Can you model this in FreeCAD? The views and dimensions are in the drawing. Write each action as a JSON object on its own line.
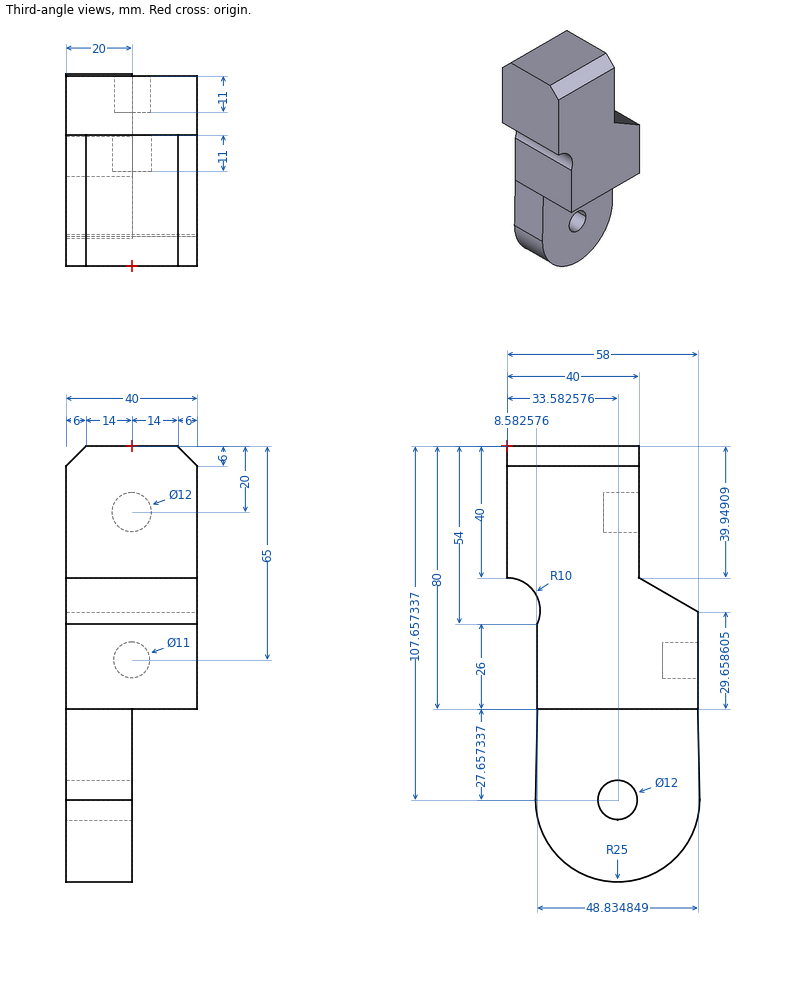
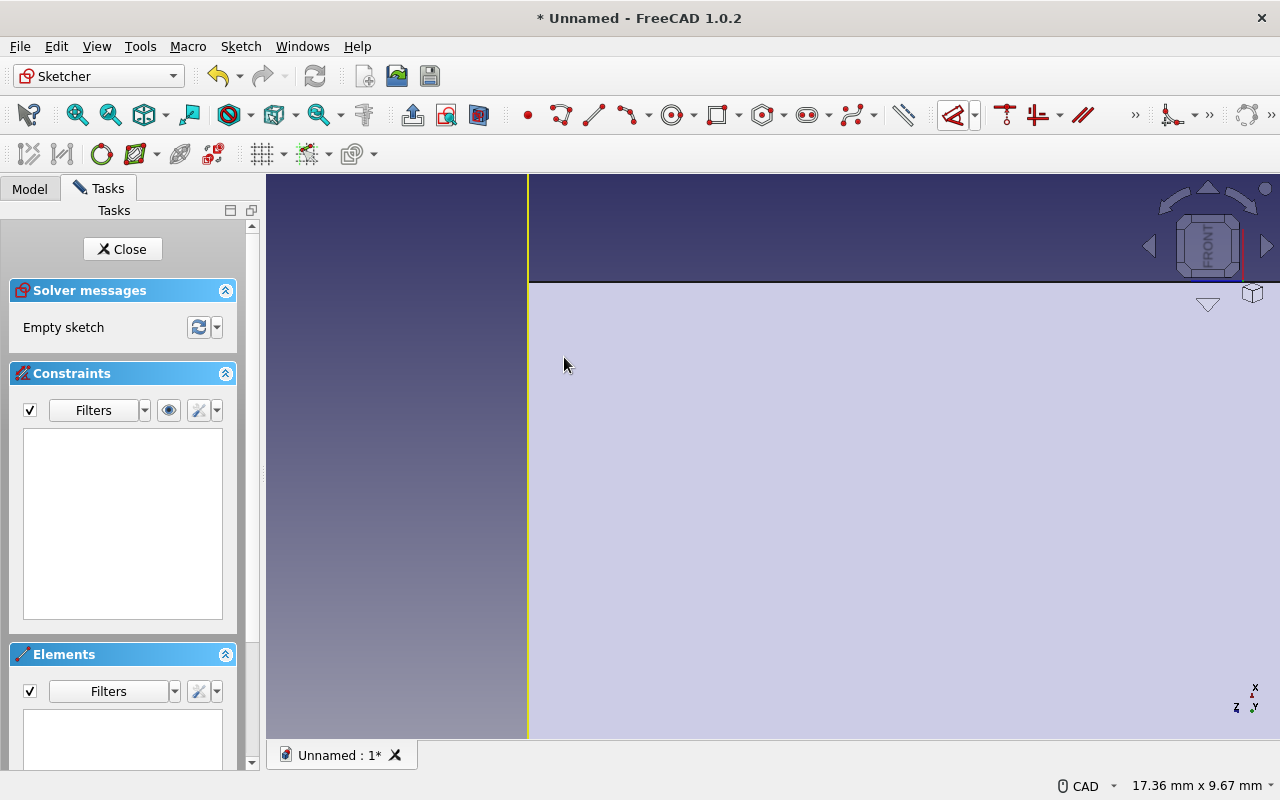
{"action": "left_click", "coordinate": [561, 116]}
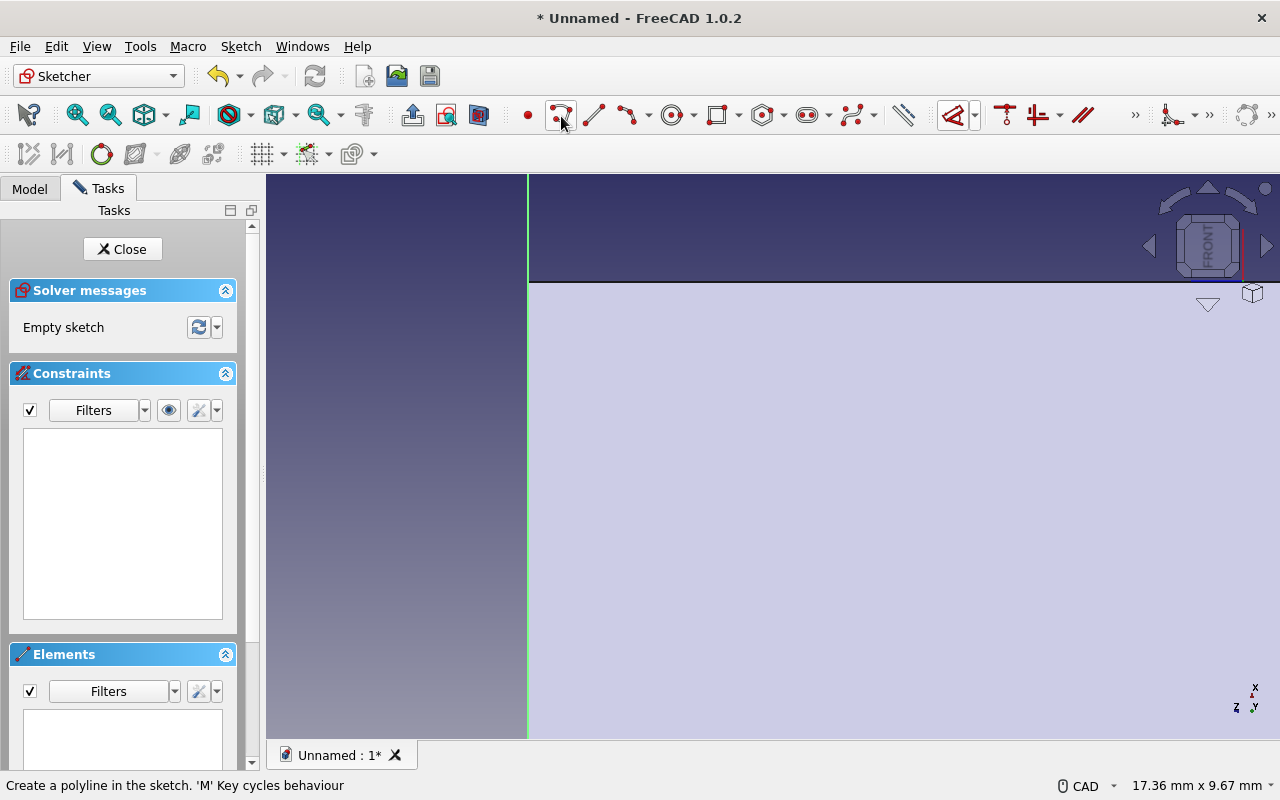
{"action": "left_click", "coordinate": [528, 633]}
{"action": "left_click", "coordinate": [878, 282]}
{"action": "left_click", "coordinate": [537, 282]}
{"action": "left_click", "coordinate": [528, 634]}
{"action": "key", "text": "Escape"}
{"action": "key", "text": "Escape"}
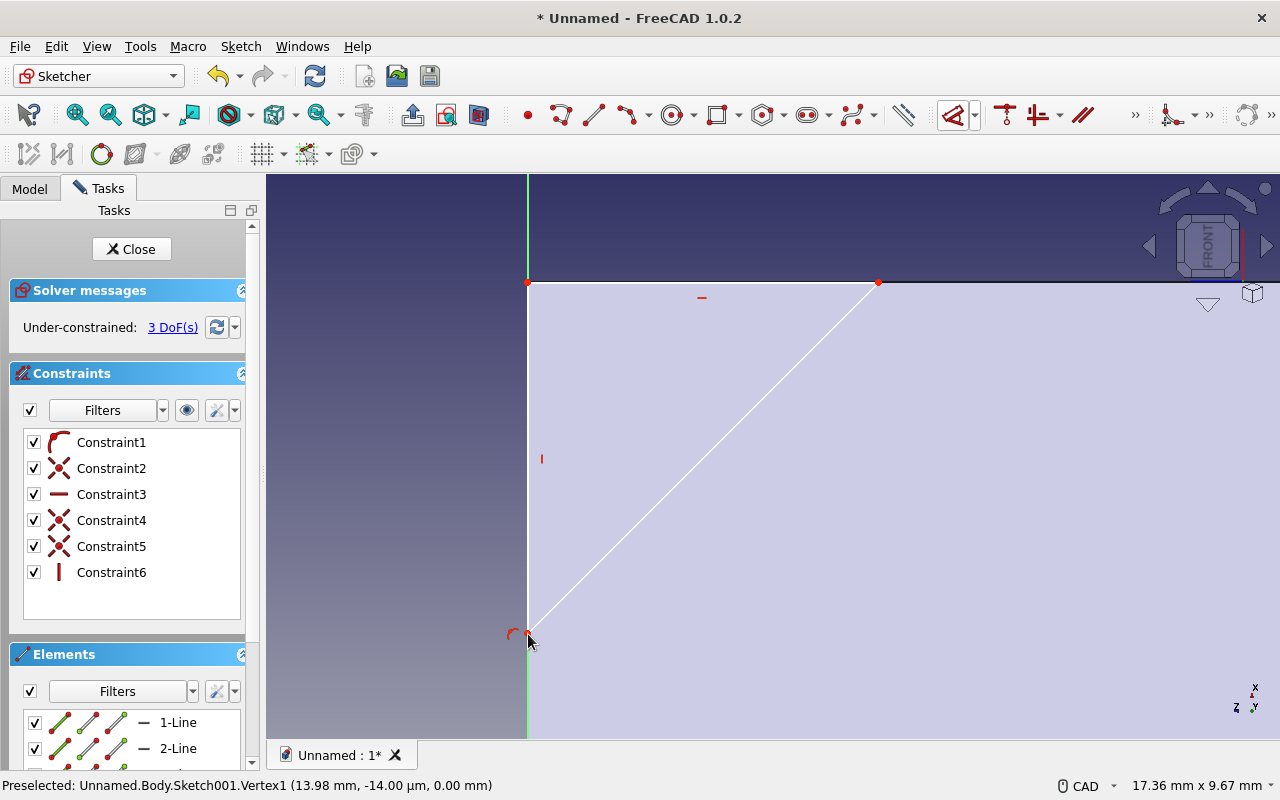
{"action": "left_click", "coordinate": [773, 283]}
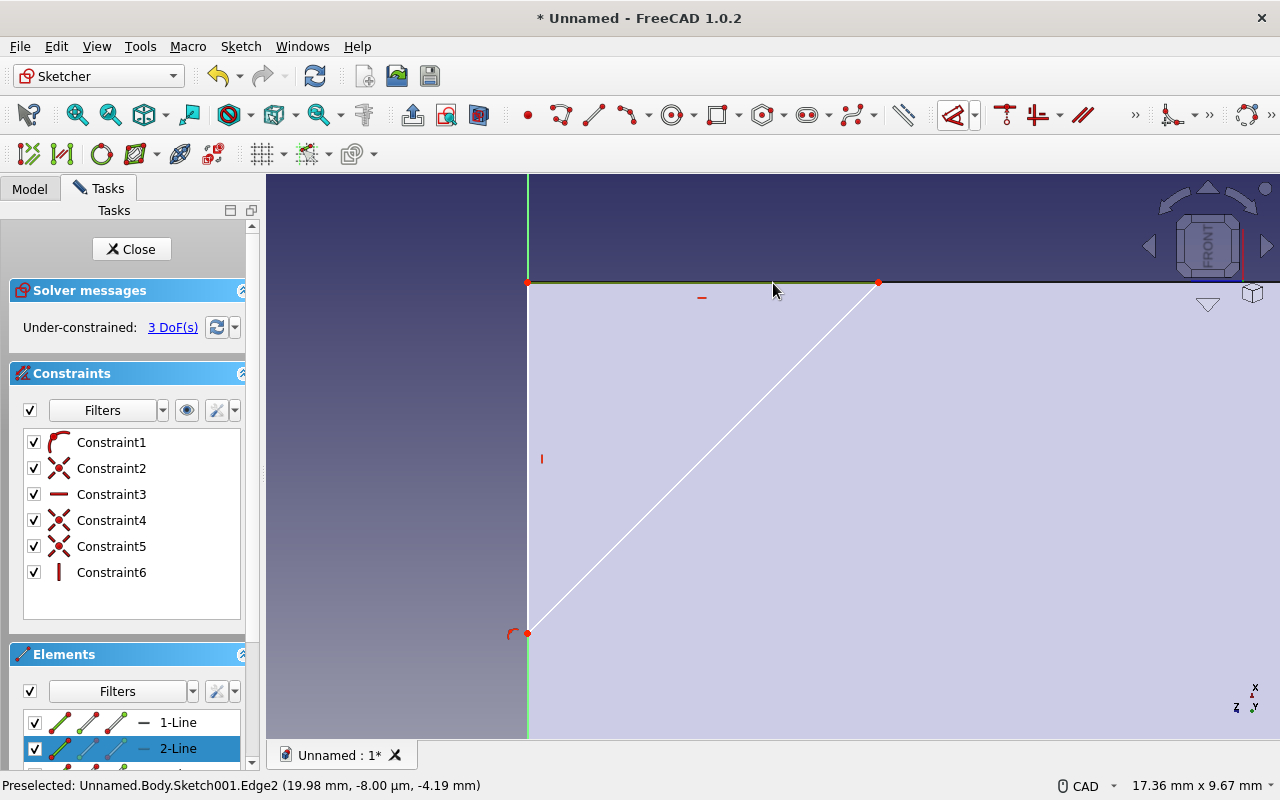
{"action": "key", "text": "l"}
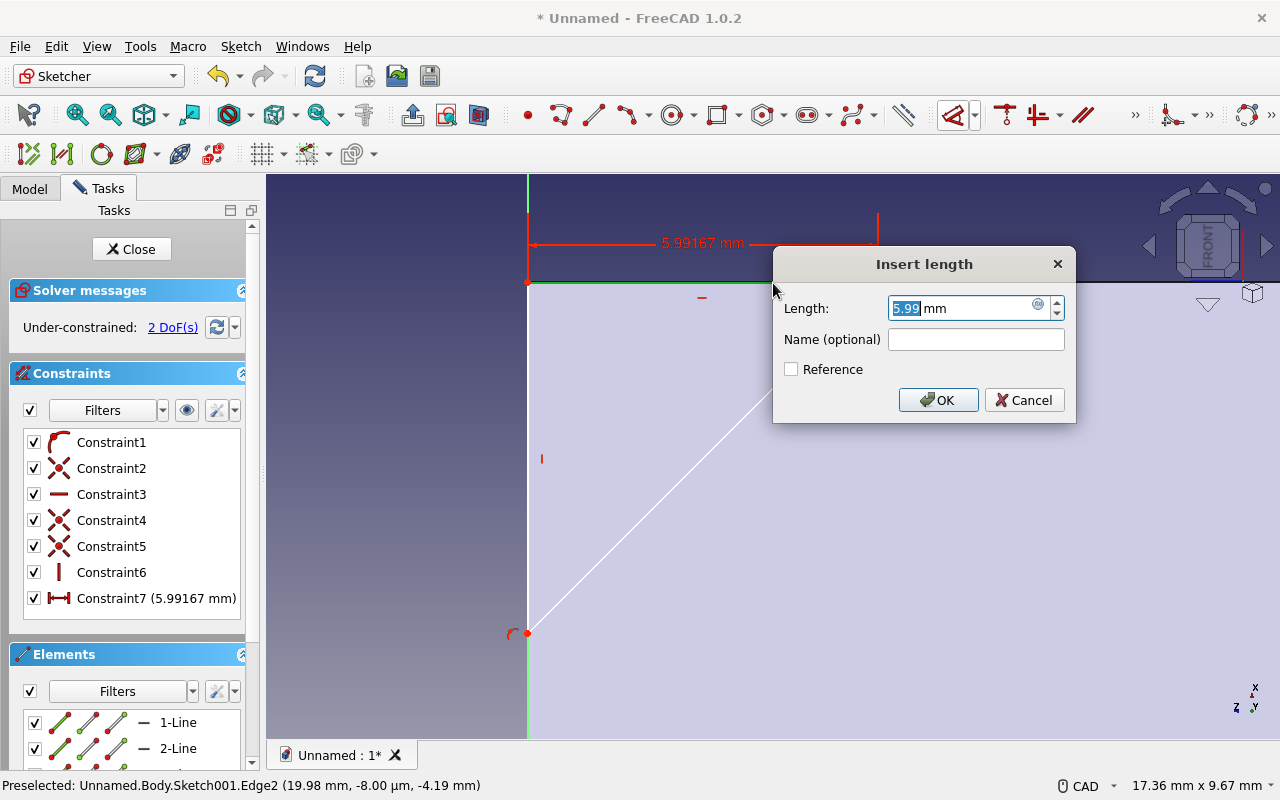
{"action": "type", "text": "6"}
{"action": "key", "text": "Return"}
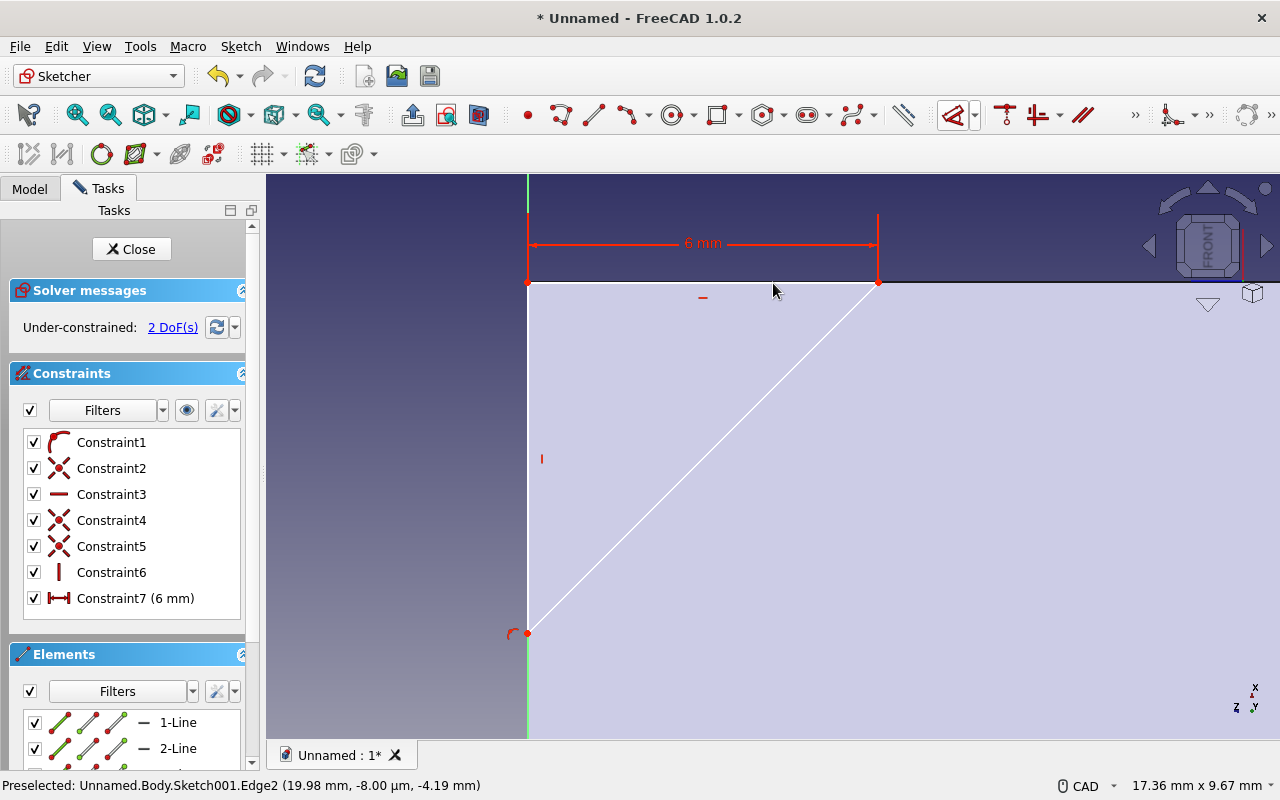
{"action": "left_click", "coordinate": [528, 388]}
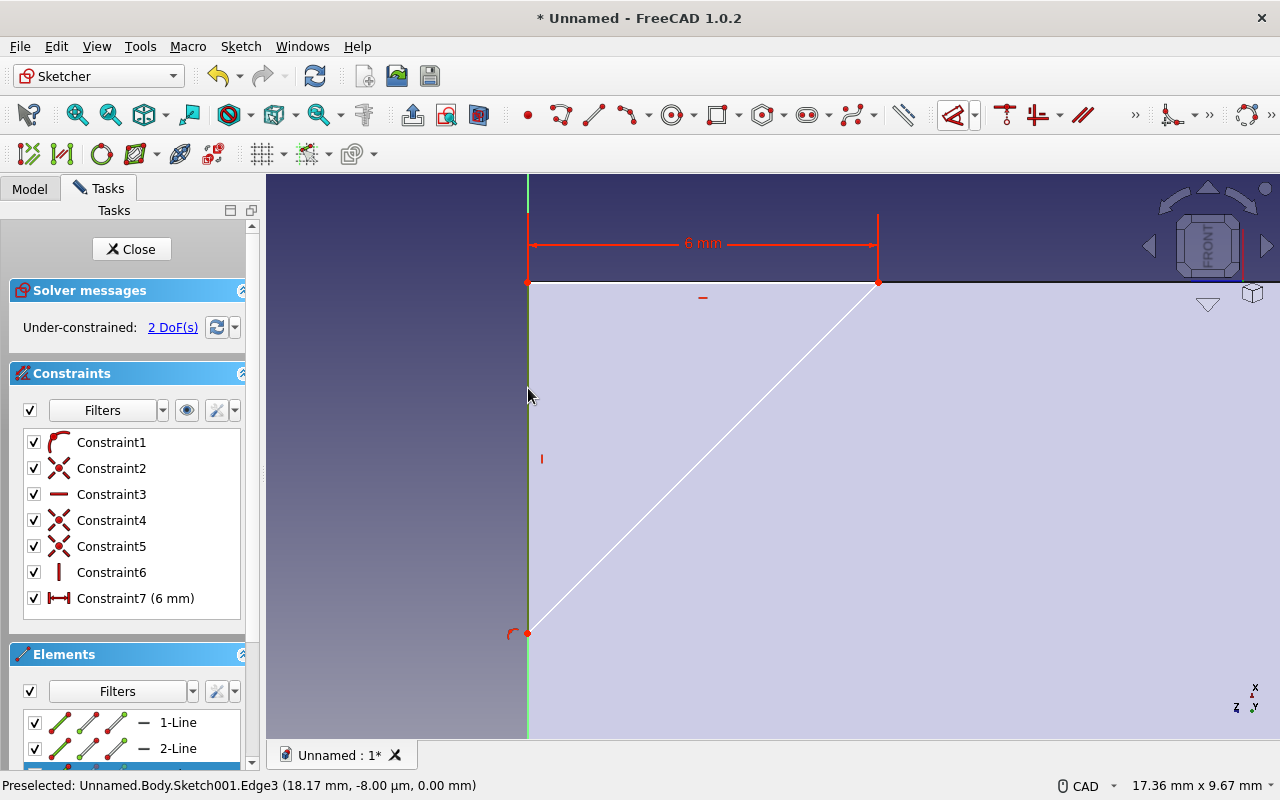
{"action": "key", "text": "i"}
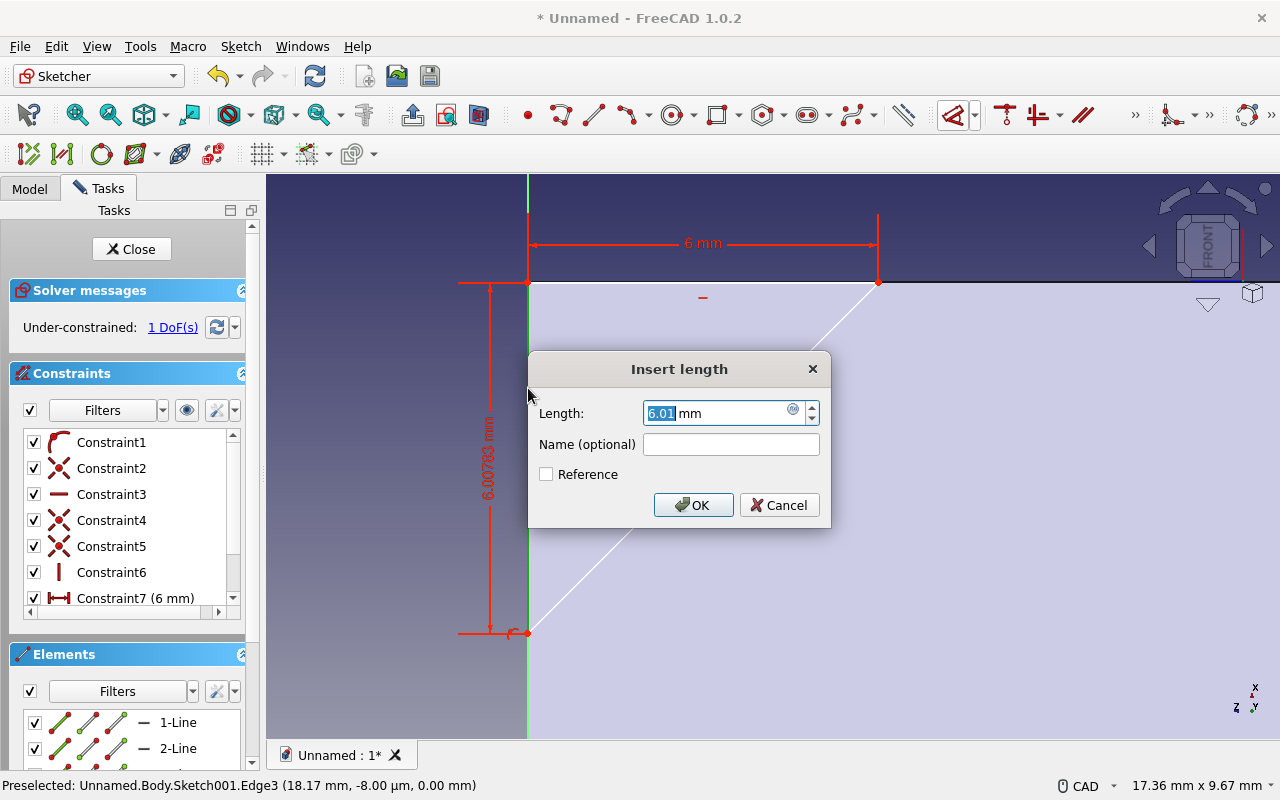
{"action": "type", "text": "6"}
{"action": "key", "text": "Return"}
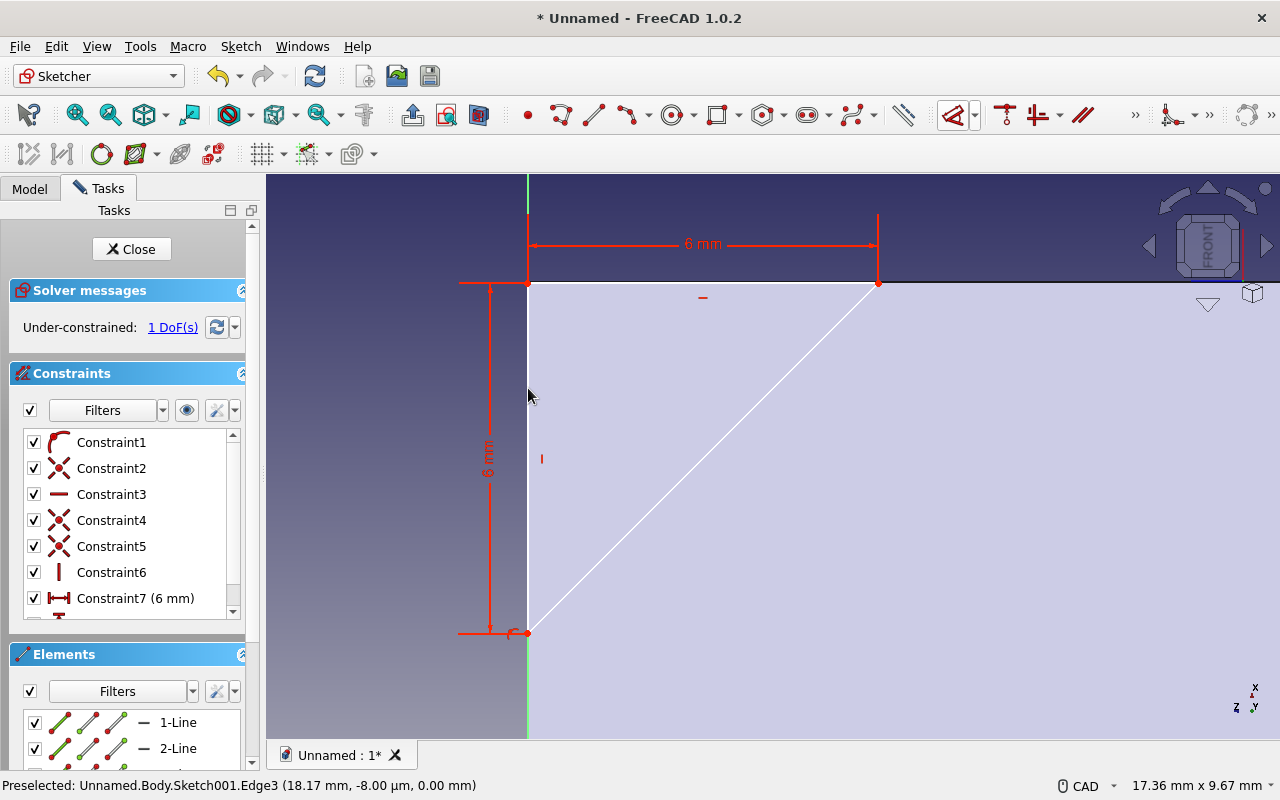
{"action": "left_click", "coordinate": [528, 634]}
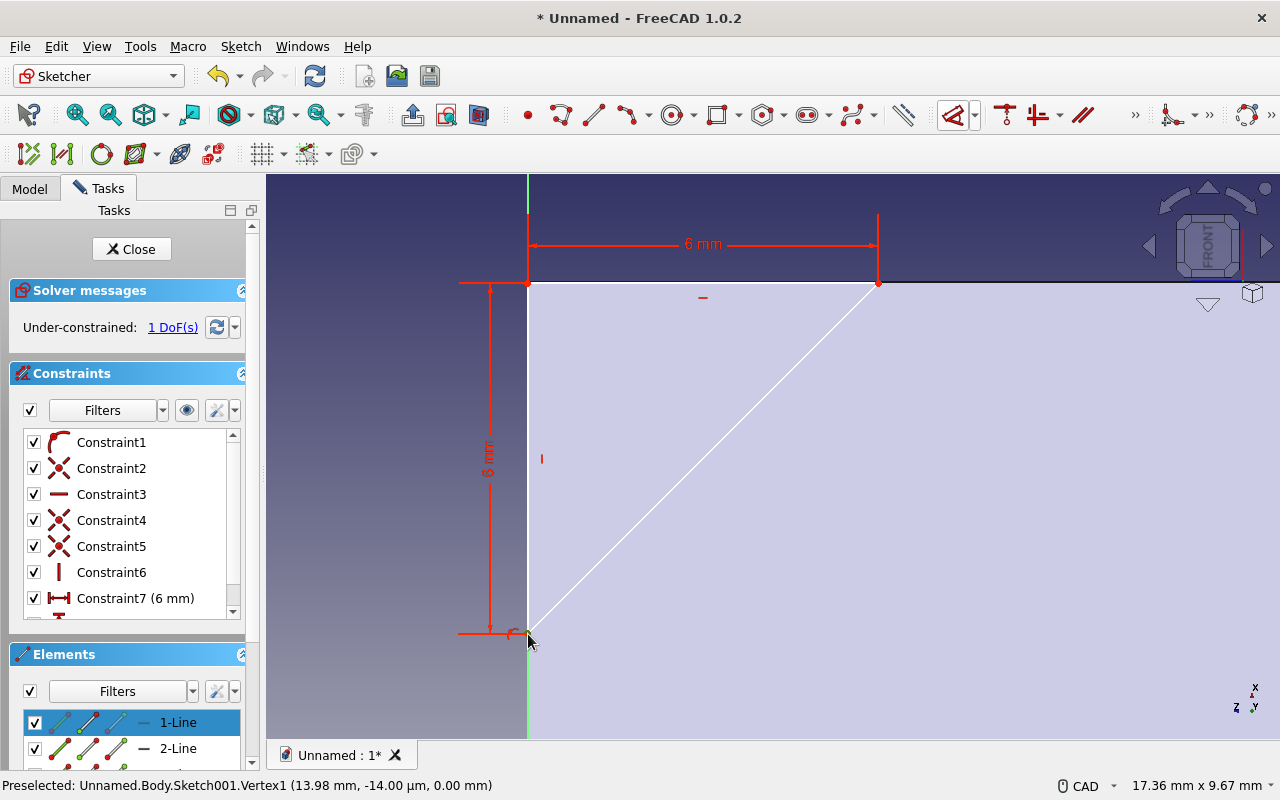
{"action": "key", "text": "i"}